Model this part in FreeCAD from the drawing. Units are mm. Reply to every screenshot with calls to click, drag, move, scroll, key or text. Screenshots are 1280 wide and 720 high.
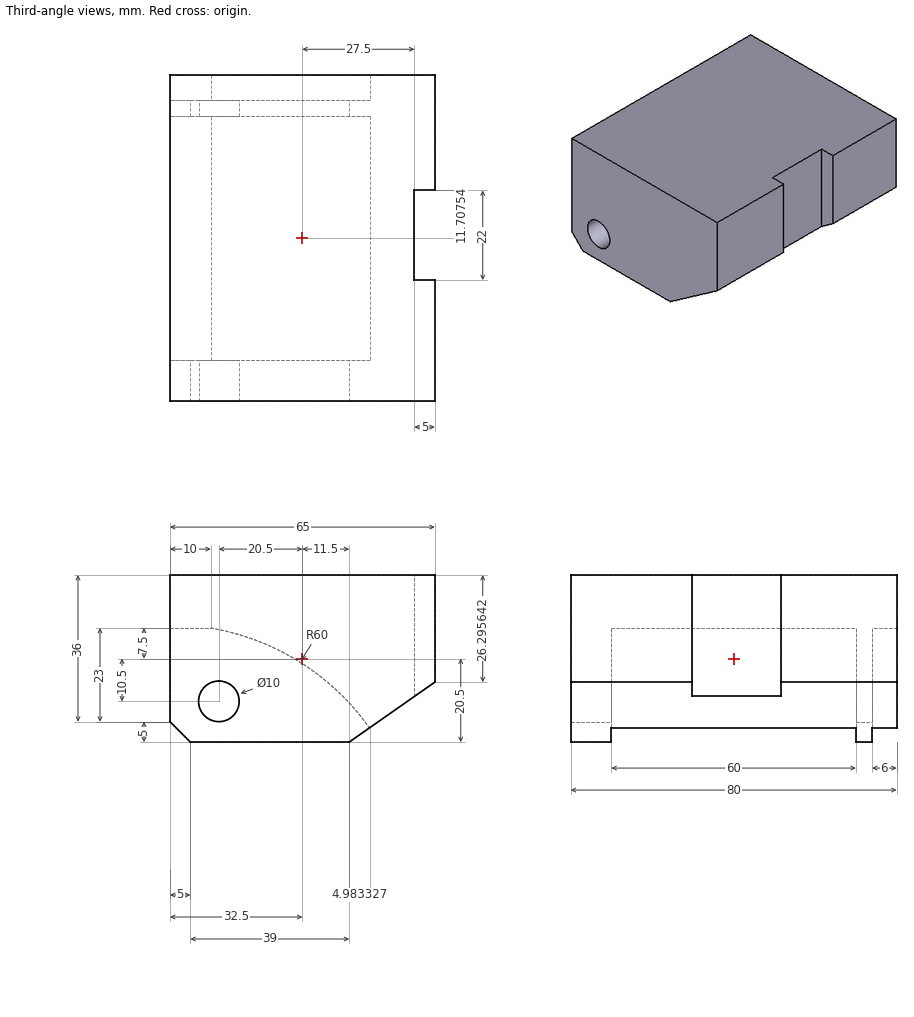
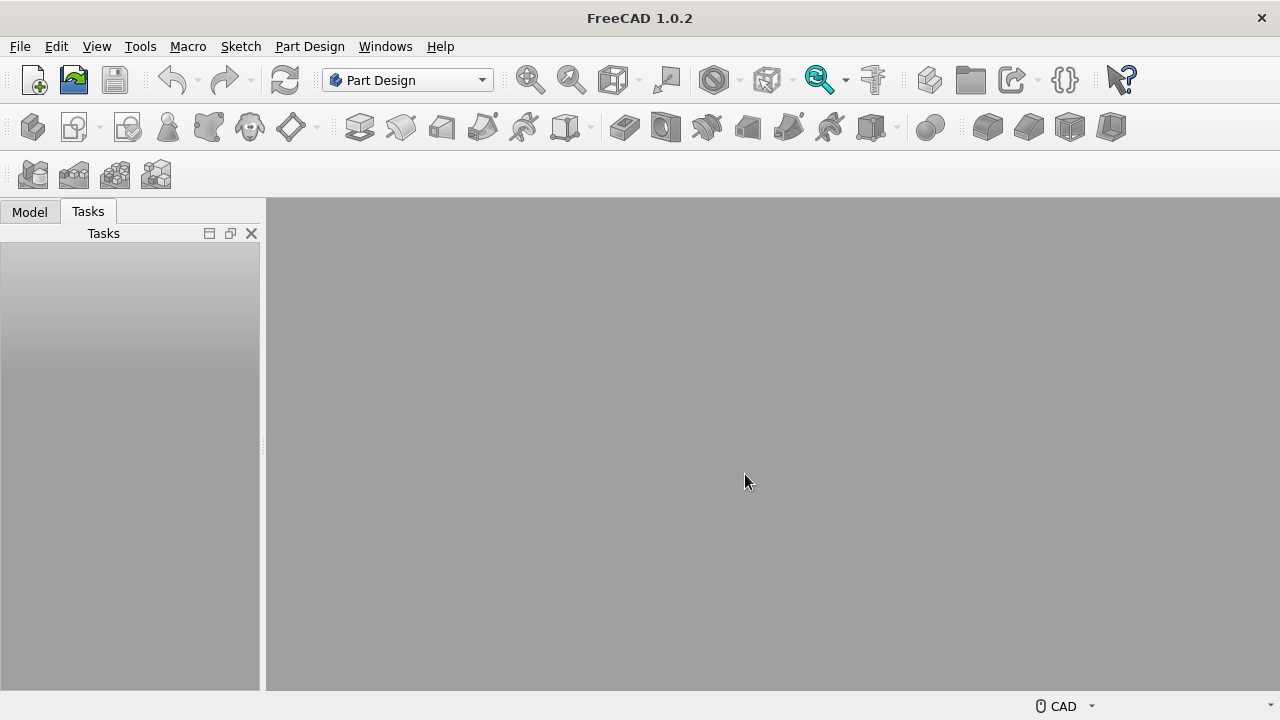
key(ctrl+n)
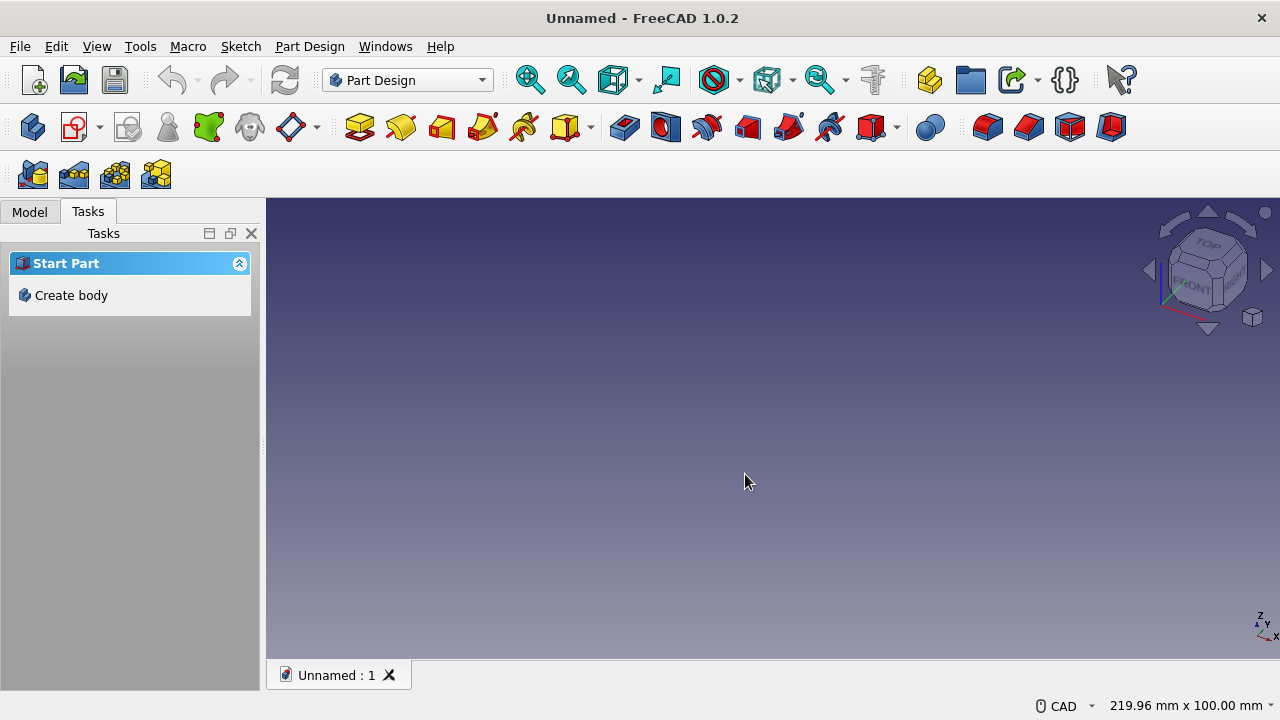
click(74, 128)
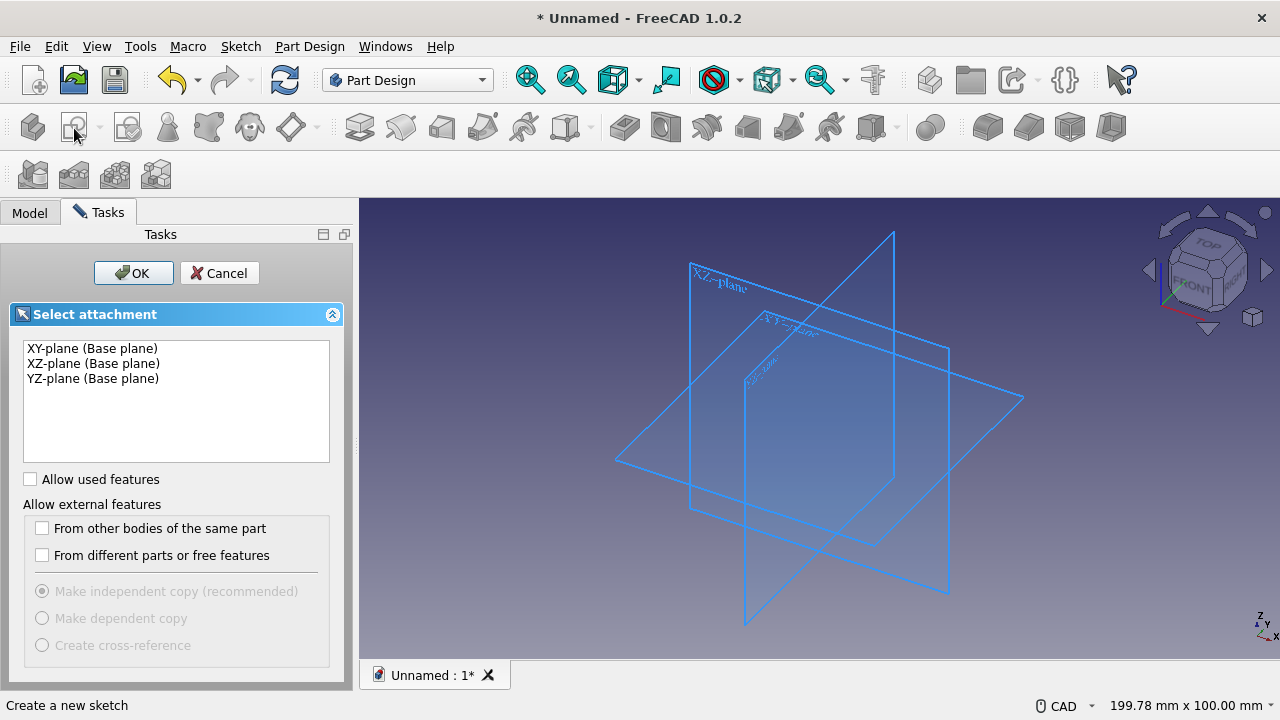
click(84, 364)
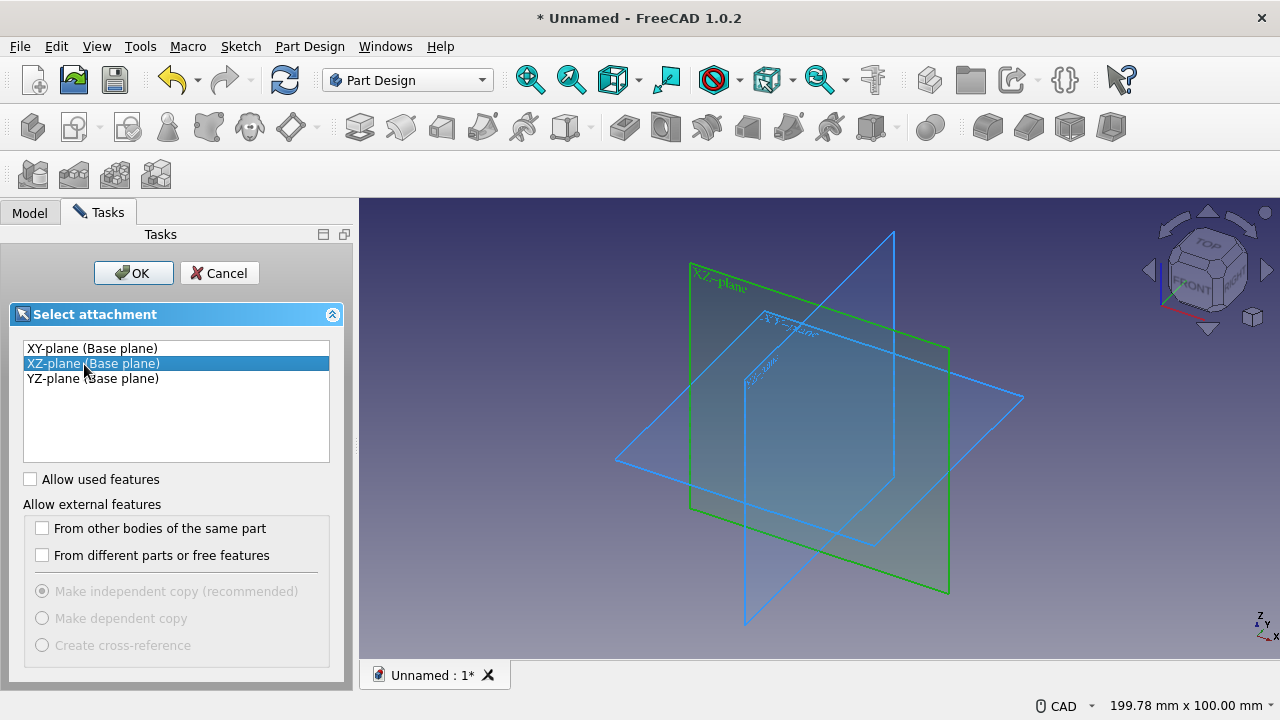
click(134, 273)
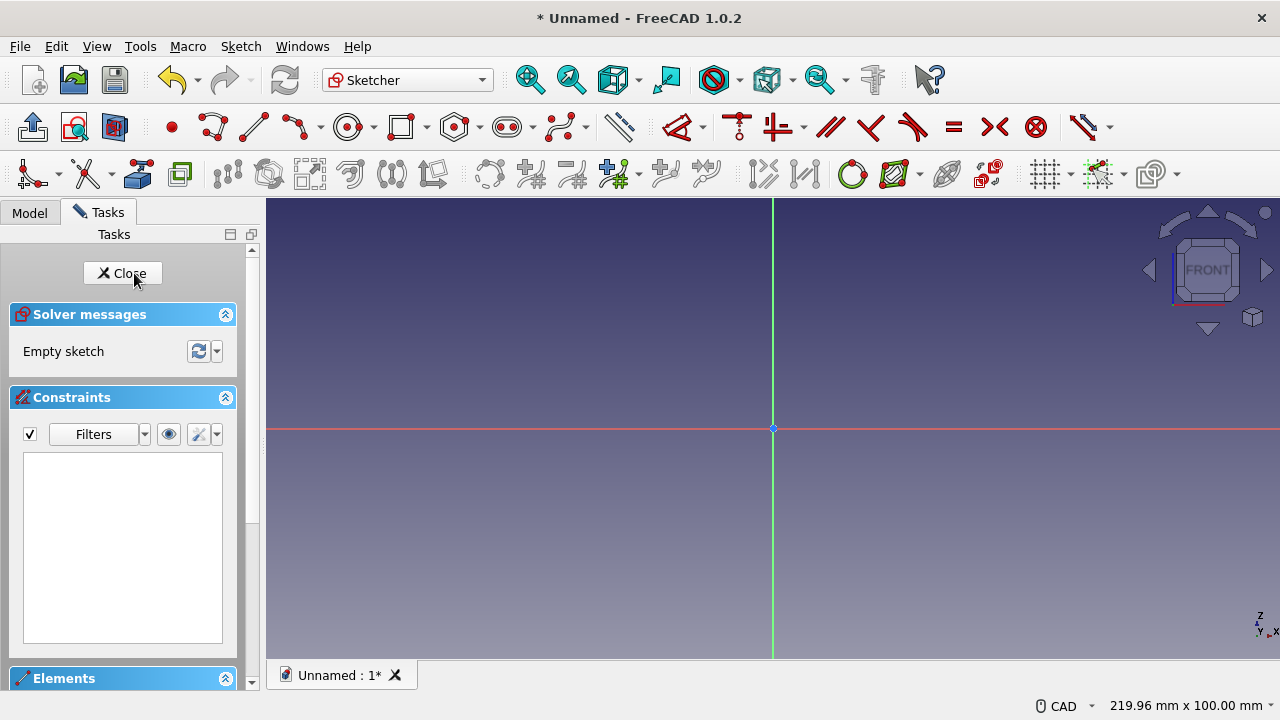
scroll(912, 428, up, 2)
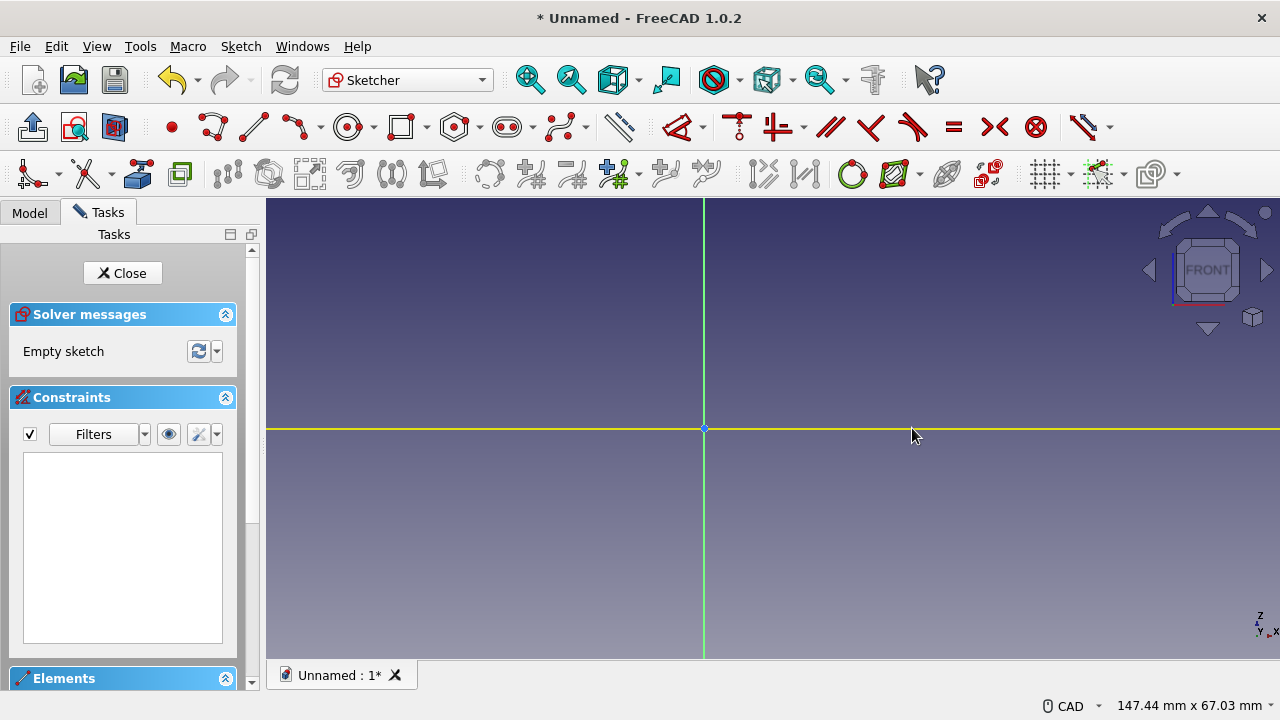
click(213, 128)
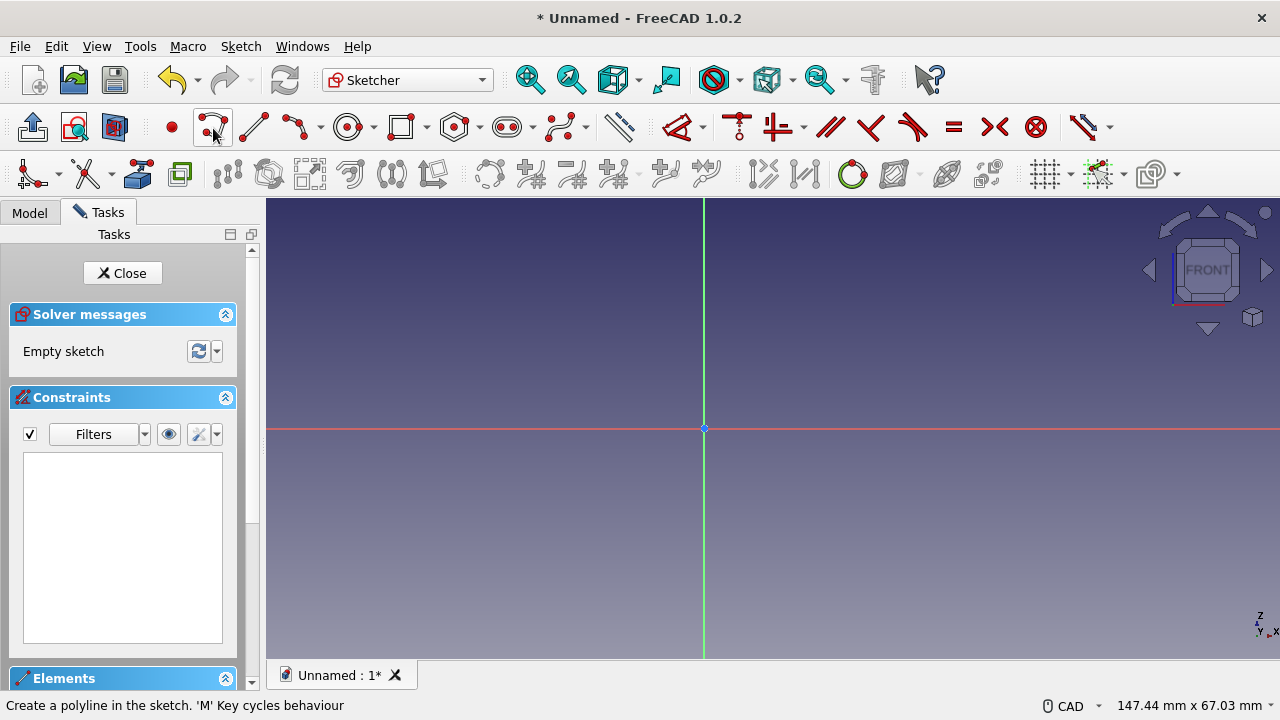
click(783, 569)
click(515, 569)
click(481, 535)
click(481, 288)
click(928, 288)
click(928, 468)
click(783, 570)
key(Escape)
key(Escape)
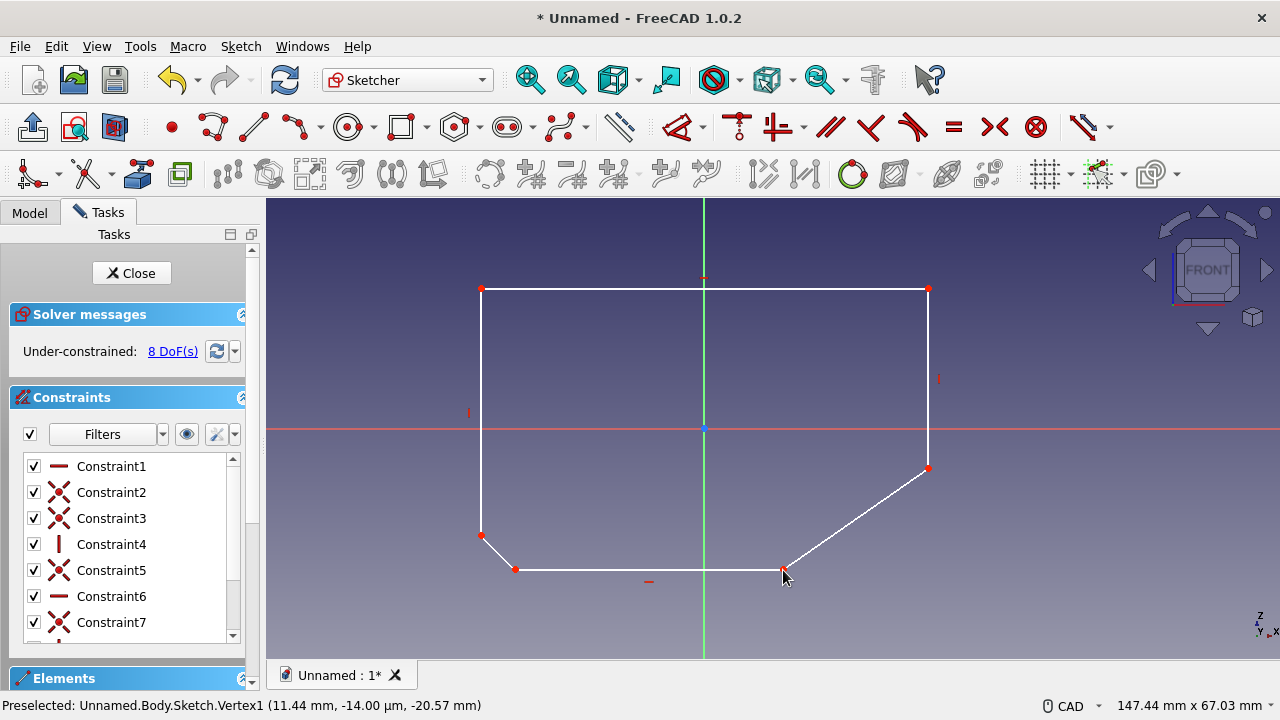
key(d)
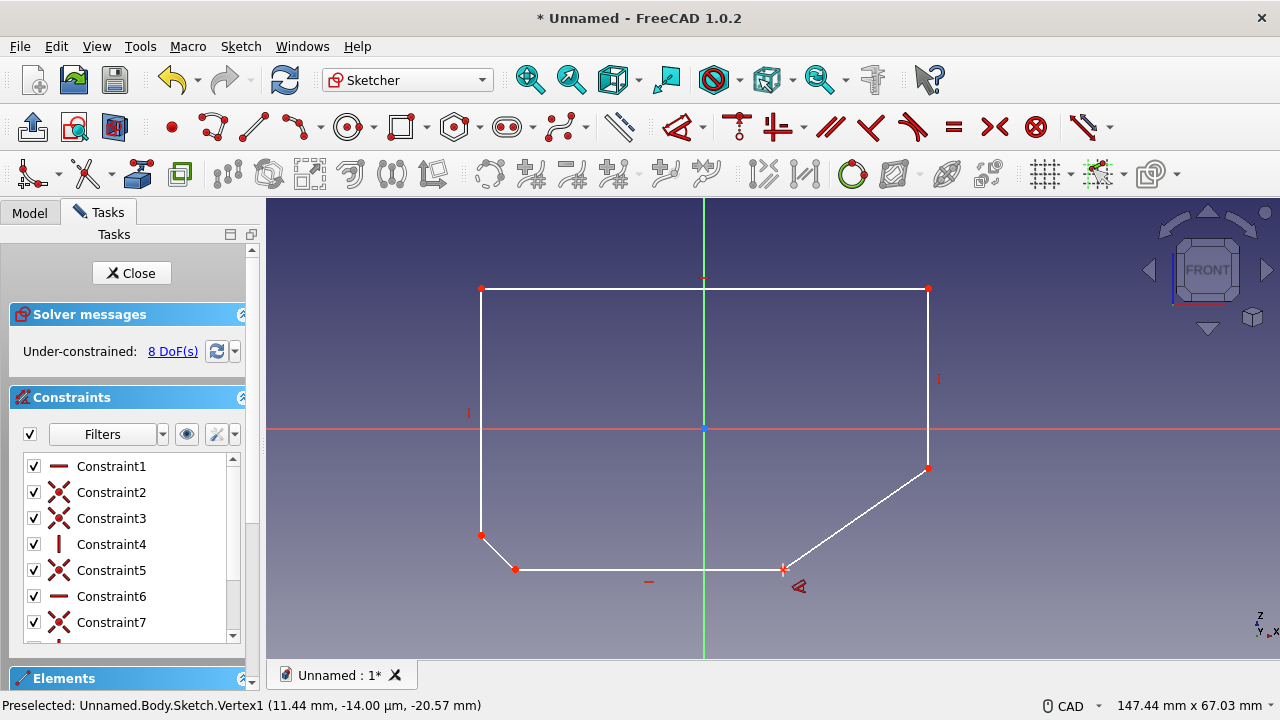
click(703, 570)
click(649, 604)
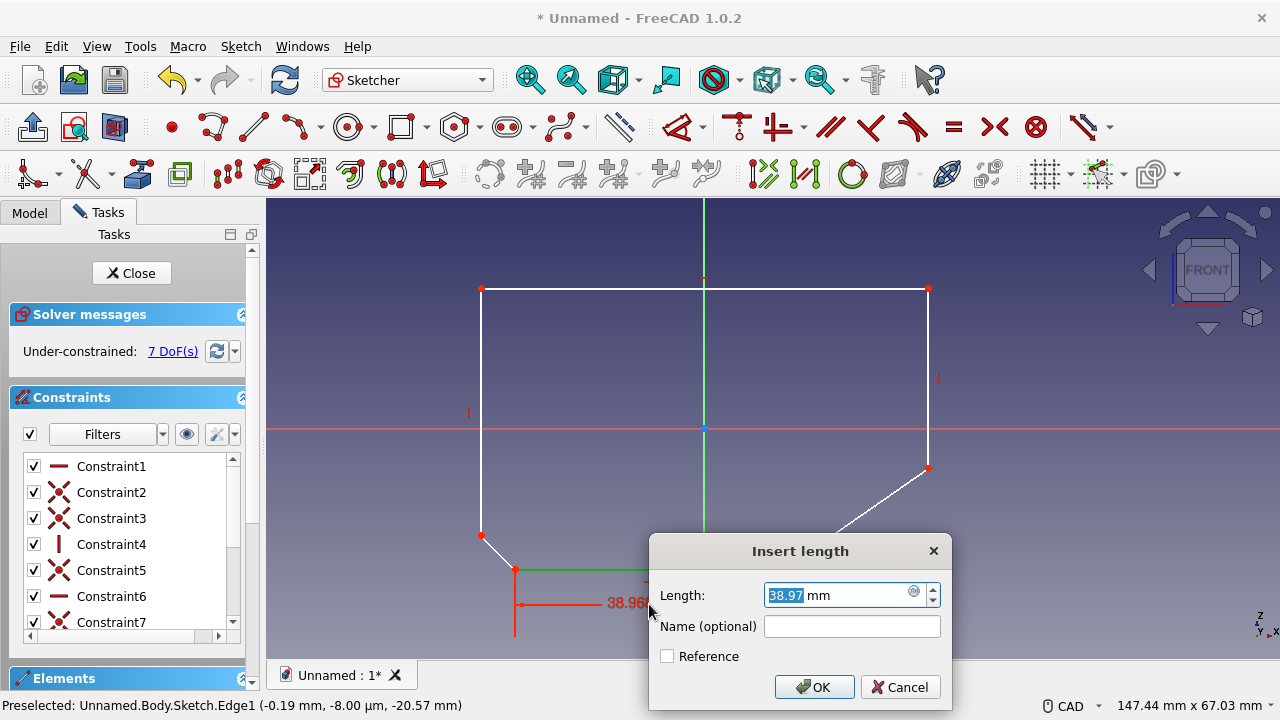
text(39)
key(Return)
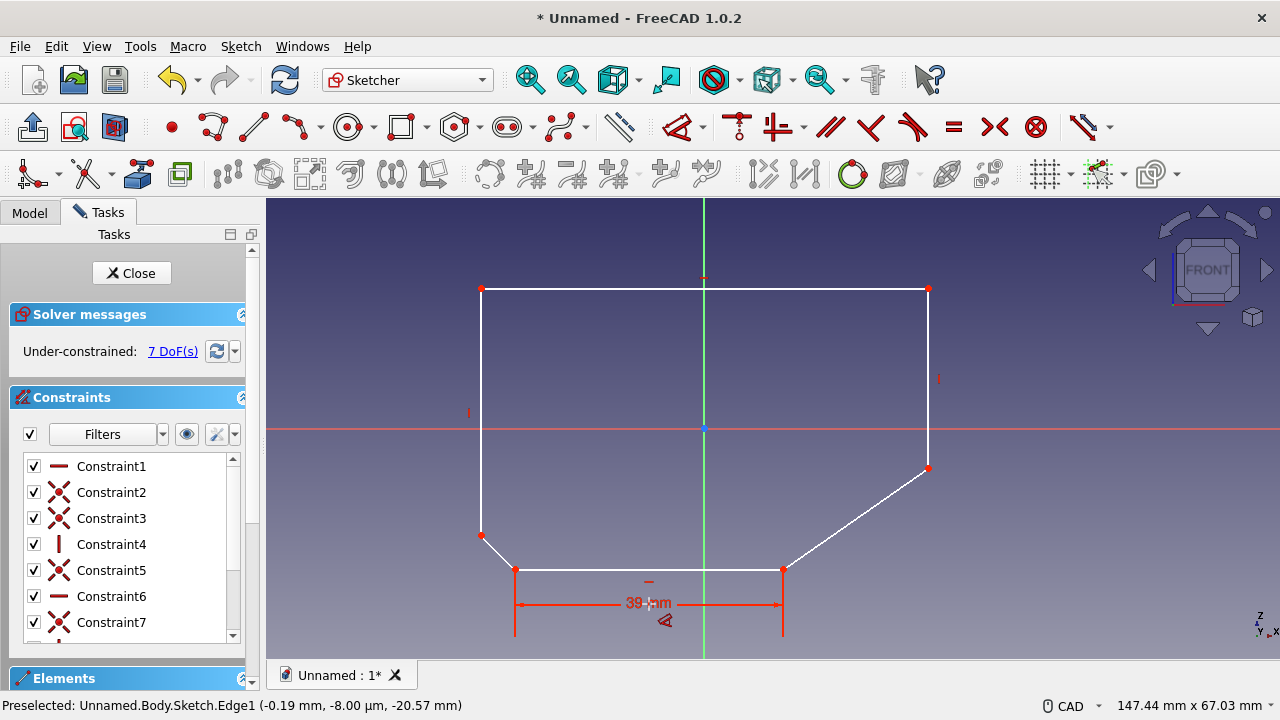
click(481, 462)
click(447, 412)